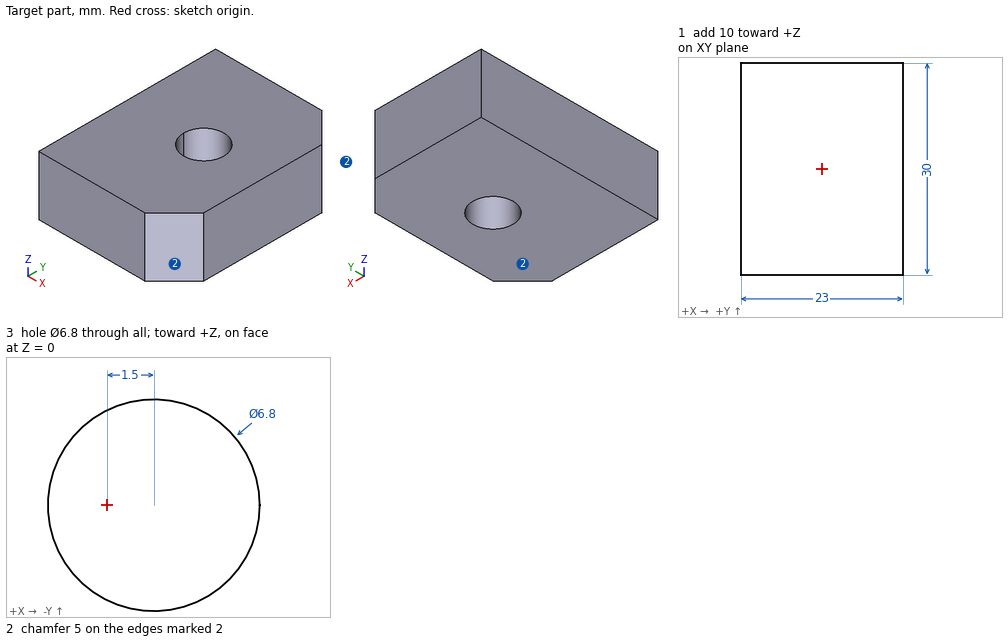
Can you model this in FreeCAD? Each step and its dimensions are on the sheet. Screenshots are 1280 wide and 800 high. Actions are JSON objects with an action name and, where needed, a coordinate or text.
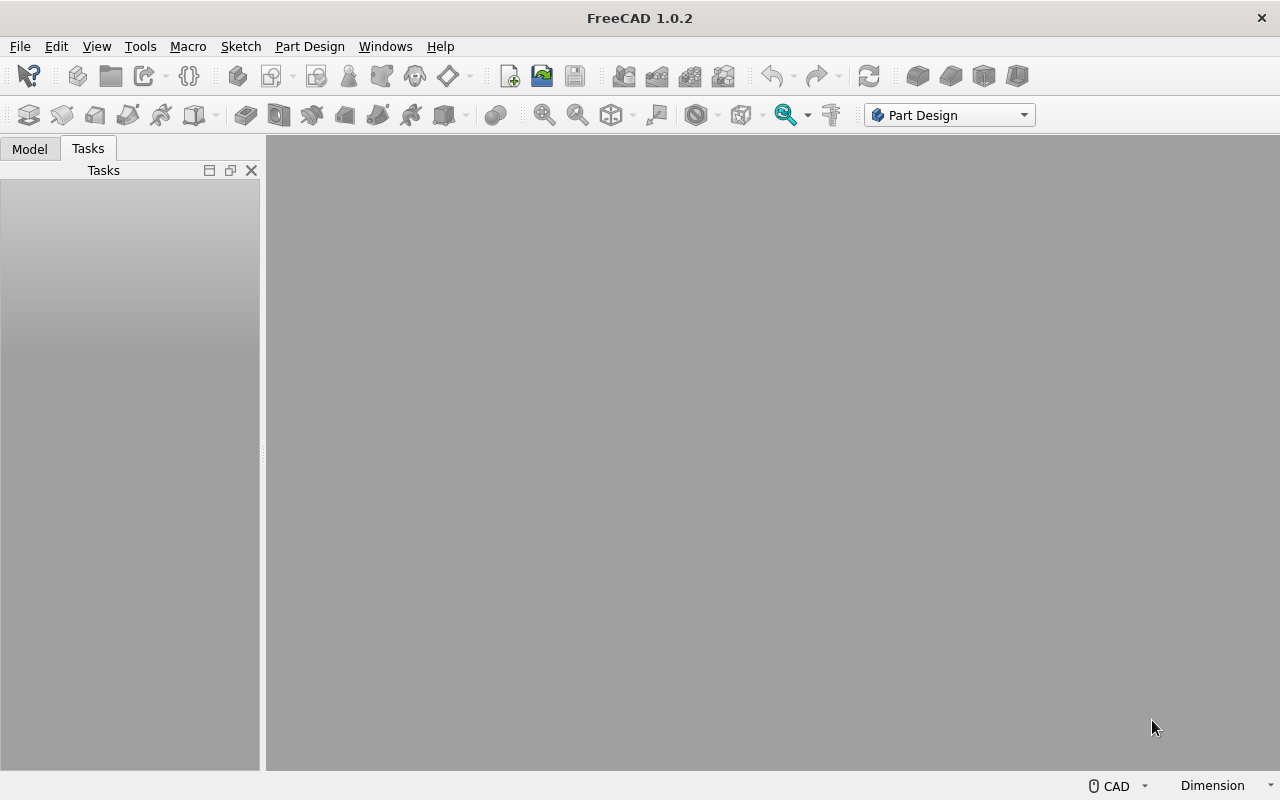
{"action": "key", "text": "ctrl+n"}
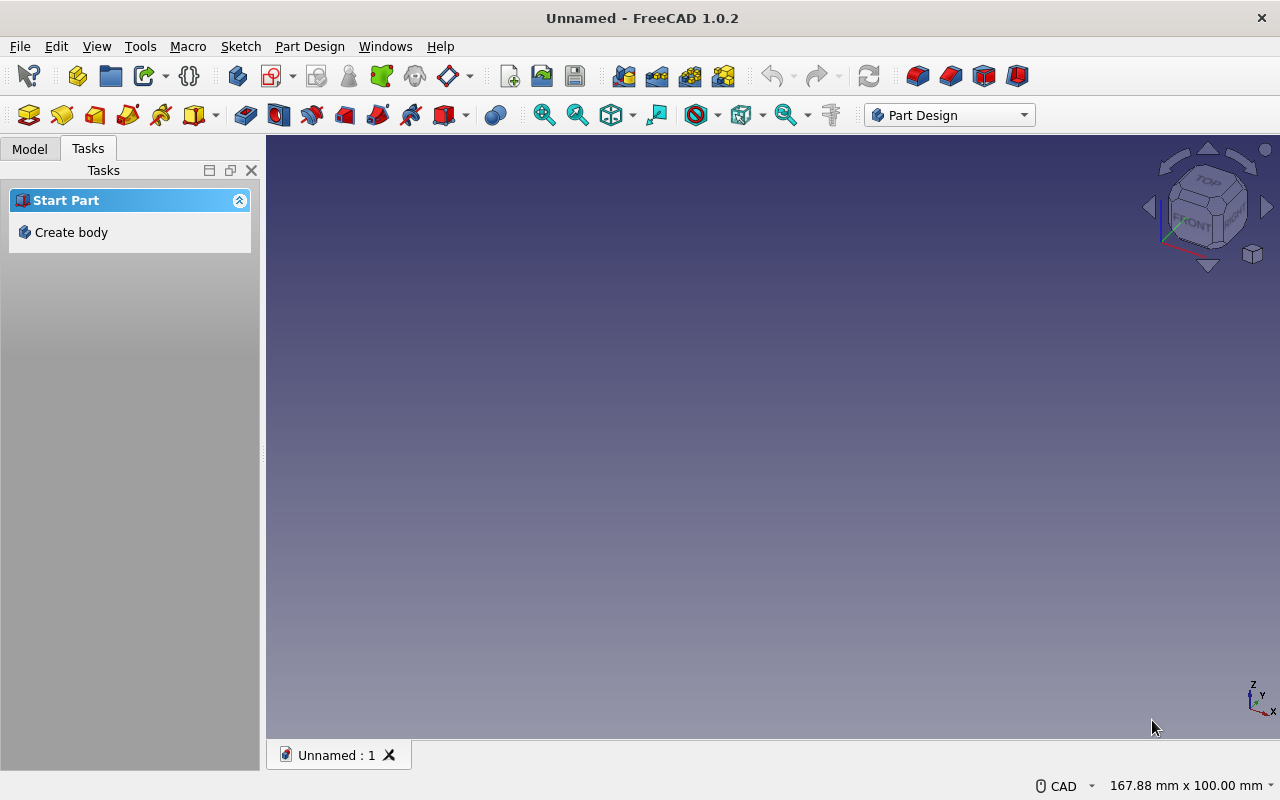
{"action": "left_click", "coordinate": [270, 76]}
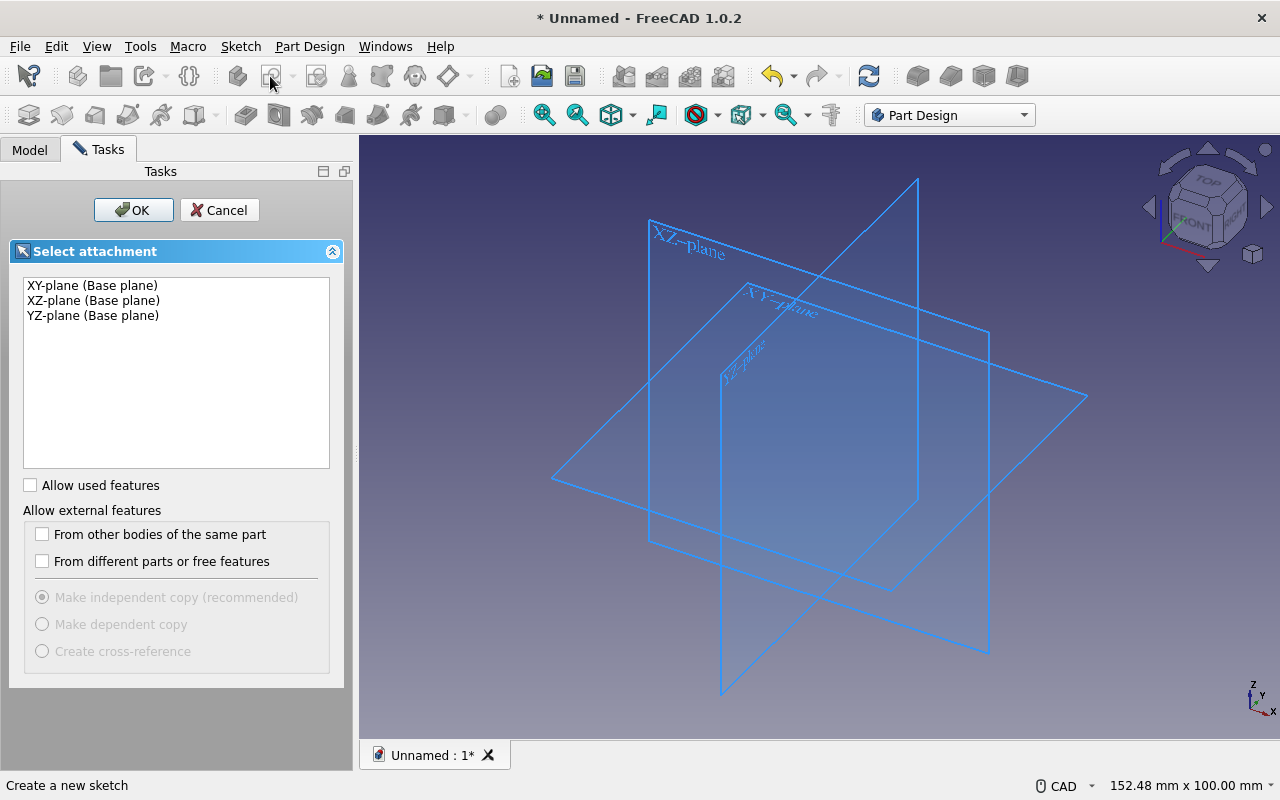
{"action": "left_click", "coordinate": [84, 286]}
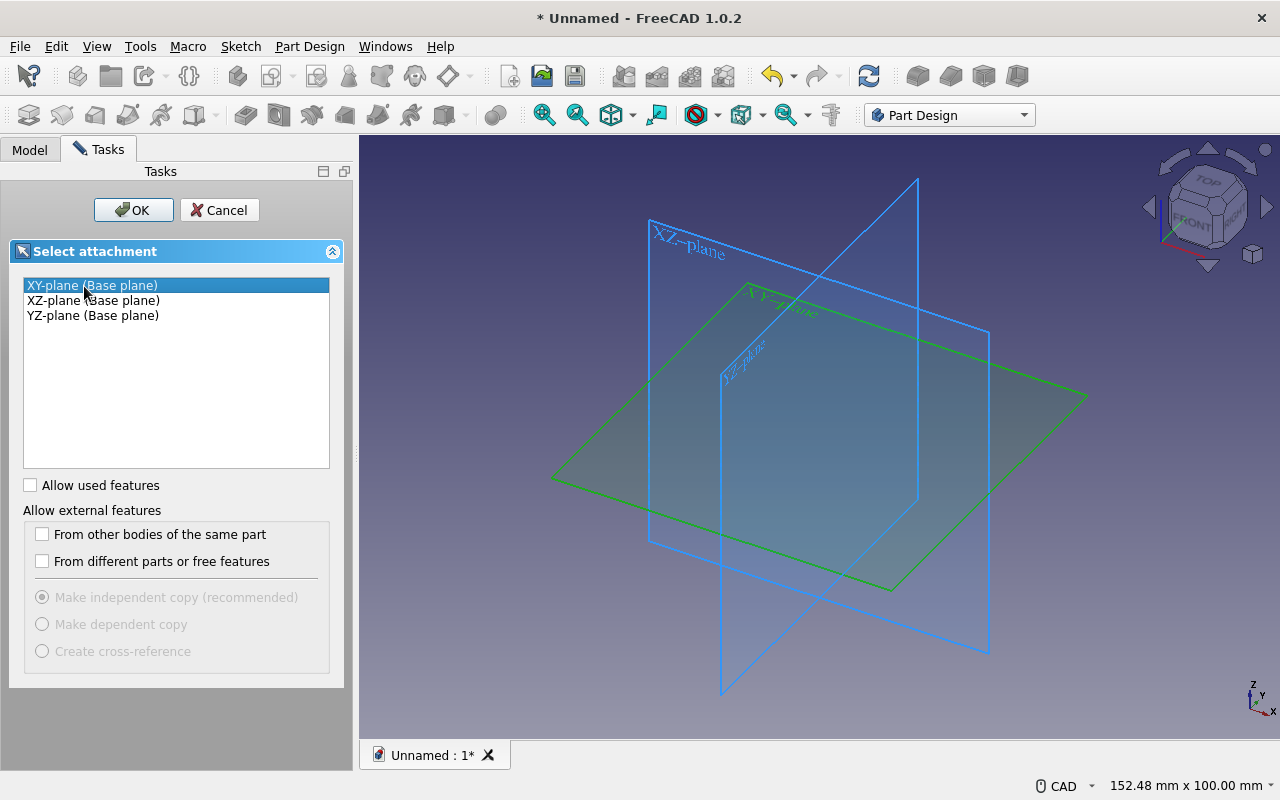
{"action": "left_click", "coordinate": [134, 210]}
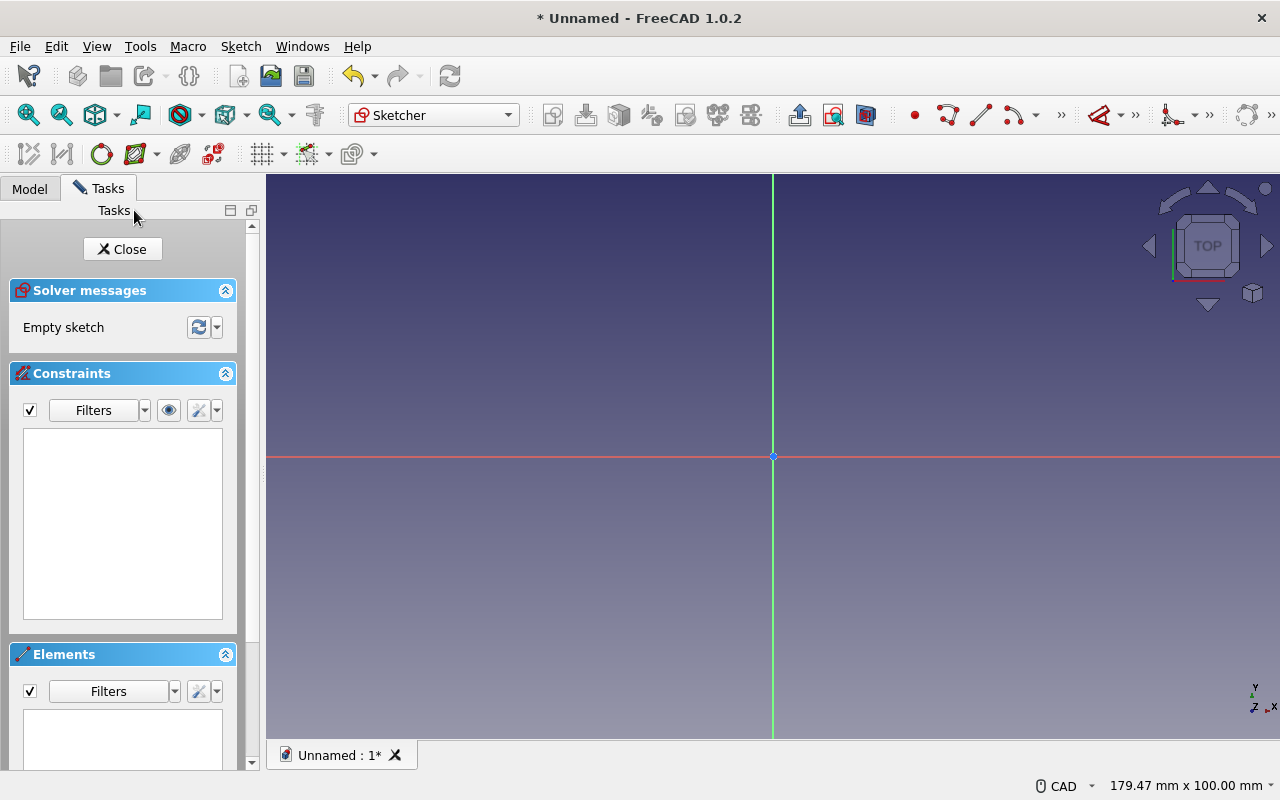
{"action": "scroll", "coordinate": [829, 456], "scroll_direction": "up", "scroll_amount": 4}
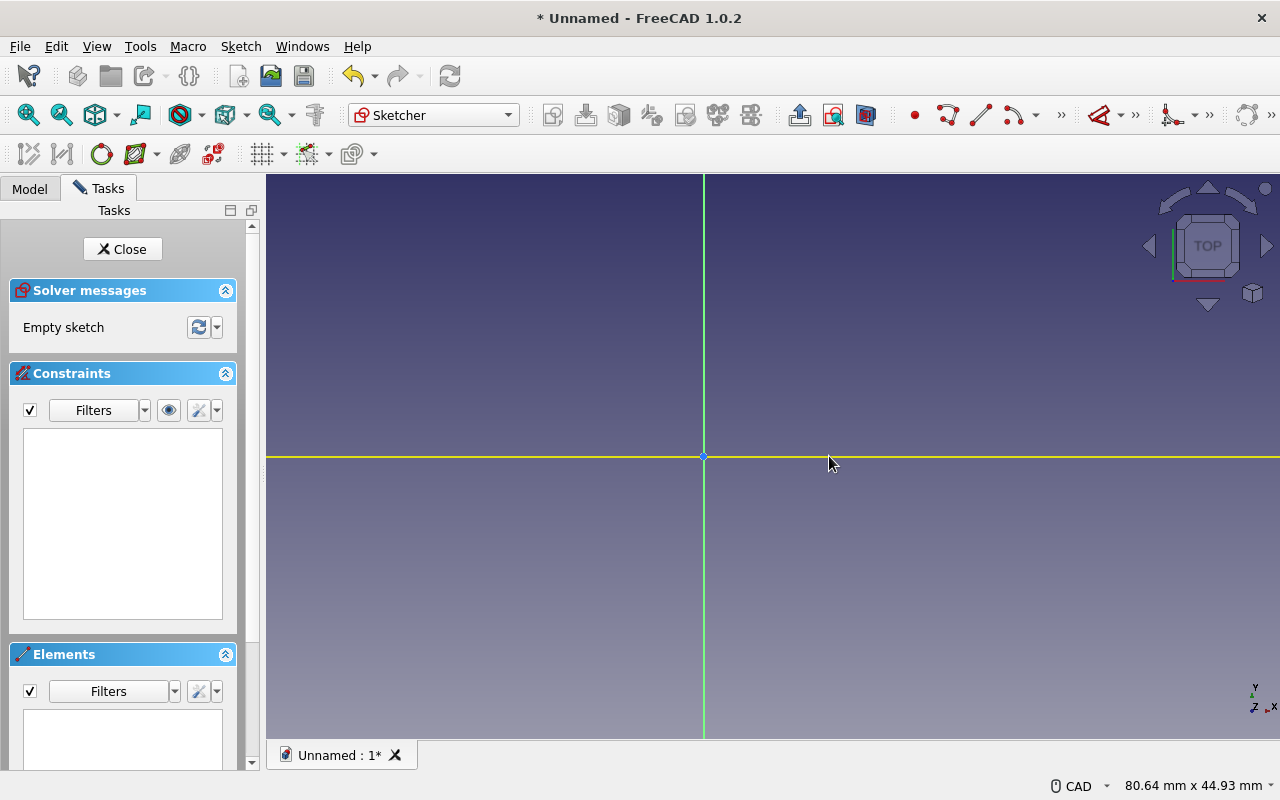
{"action": "key", "text": "g v"}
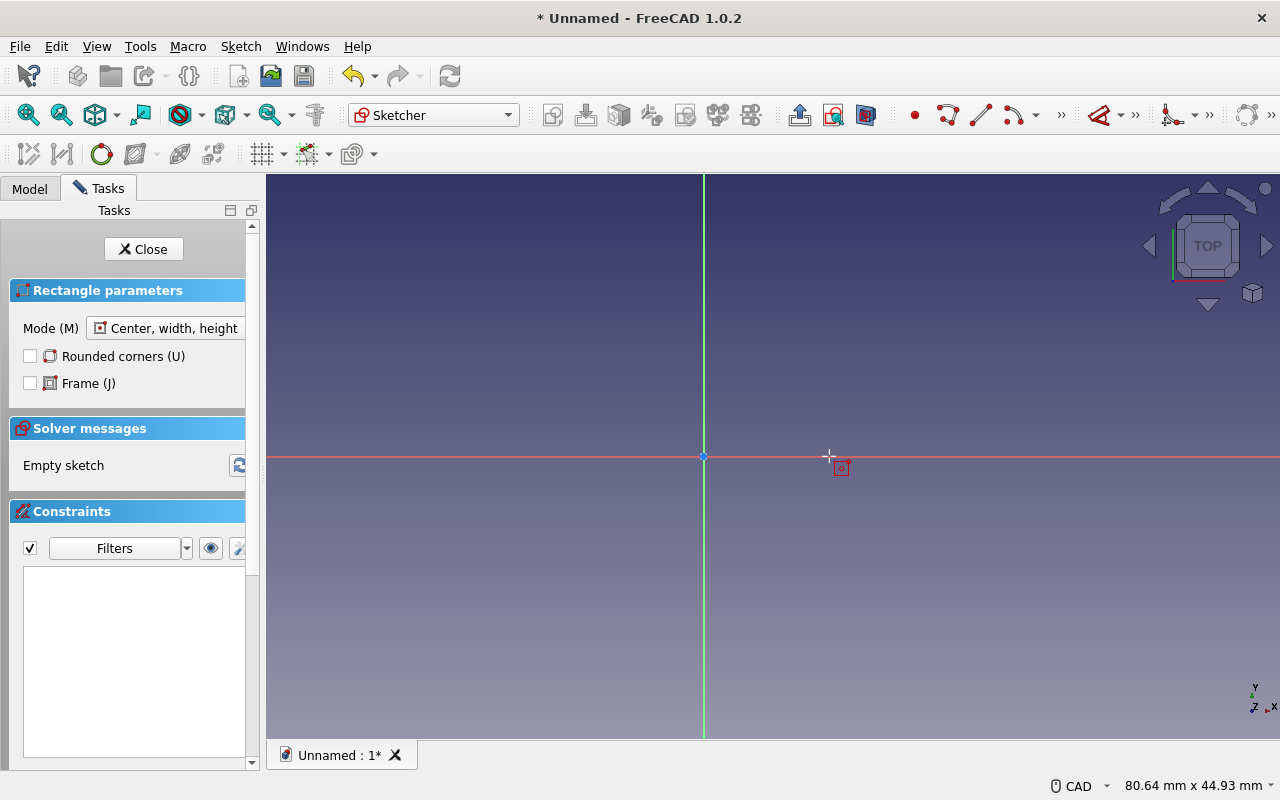
{"action": "left_click", "coordinate": [704, 456]}
{"action": "left_click", "coordinate": [848, 268]}
{"action": "key", "text": "Escape"}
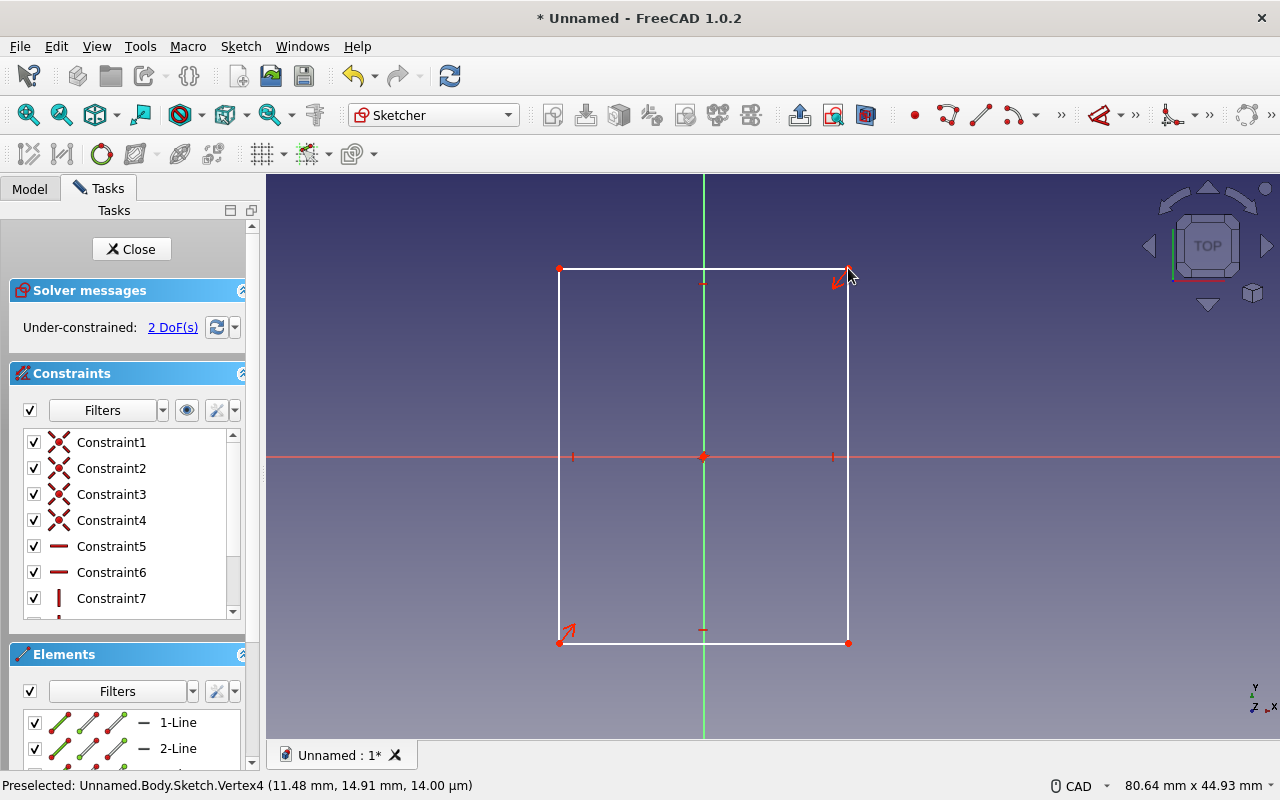
{"action": "left_click", "coordinate": [1098, 116]}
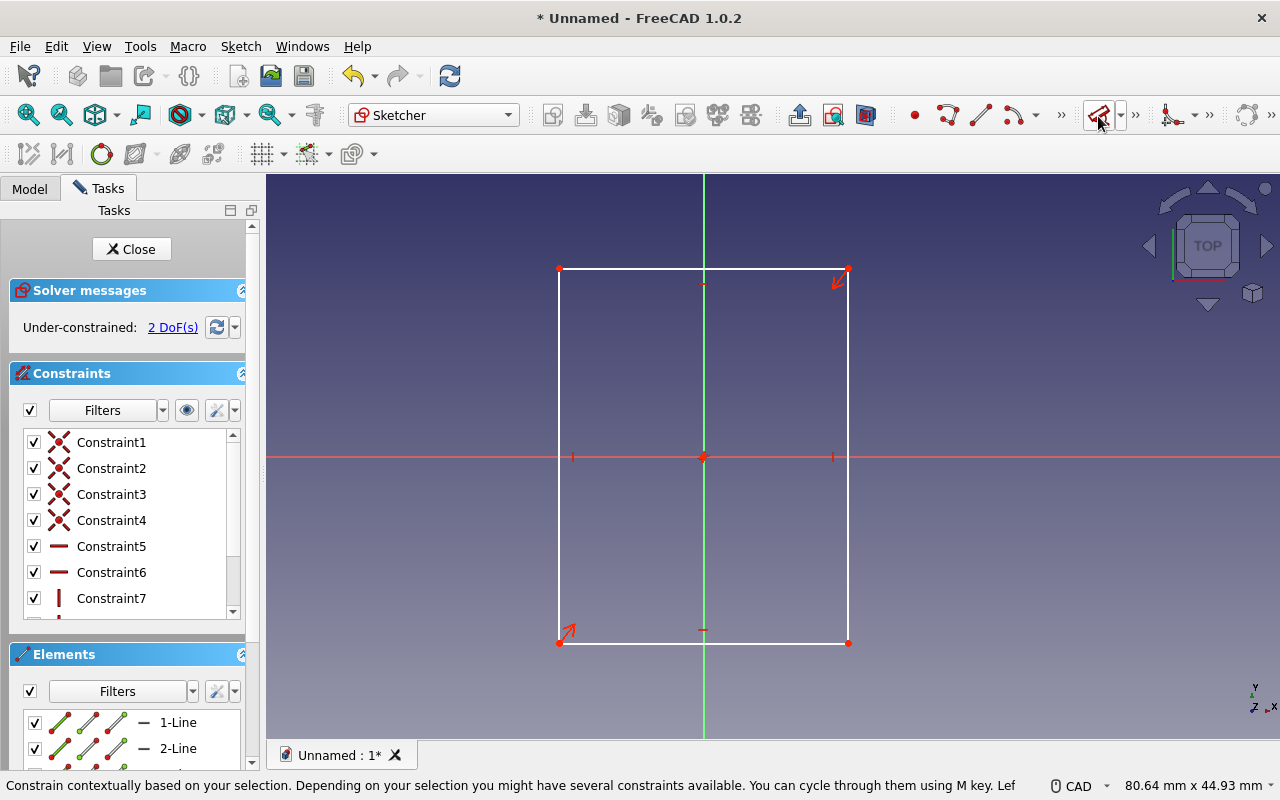
{"action": "left_click", "coordinate": [646, 644]}
{"action": "left_click", "coordinate": [637, 678]}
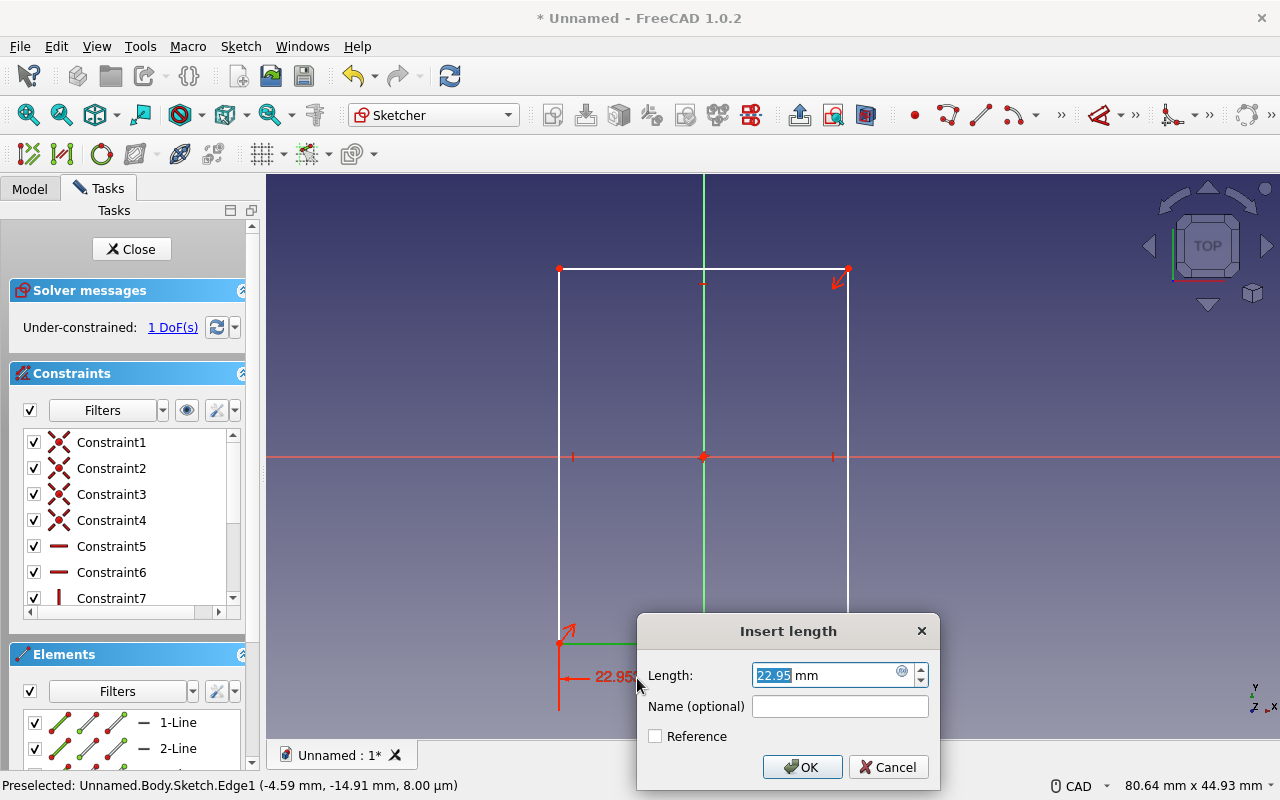
{"action": "type", "text": "23"}
{"action": "key", "text": "Return"}